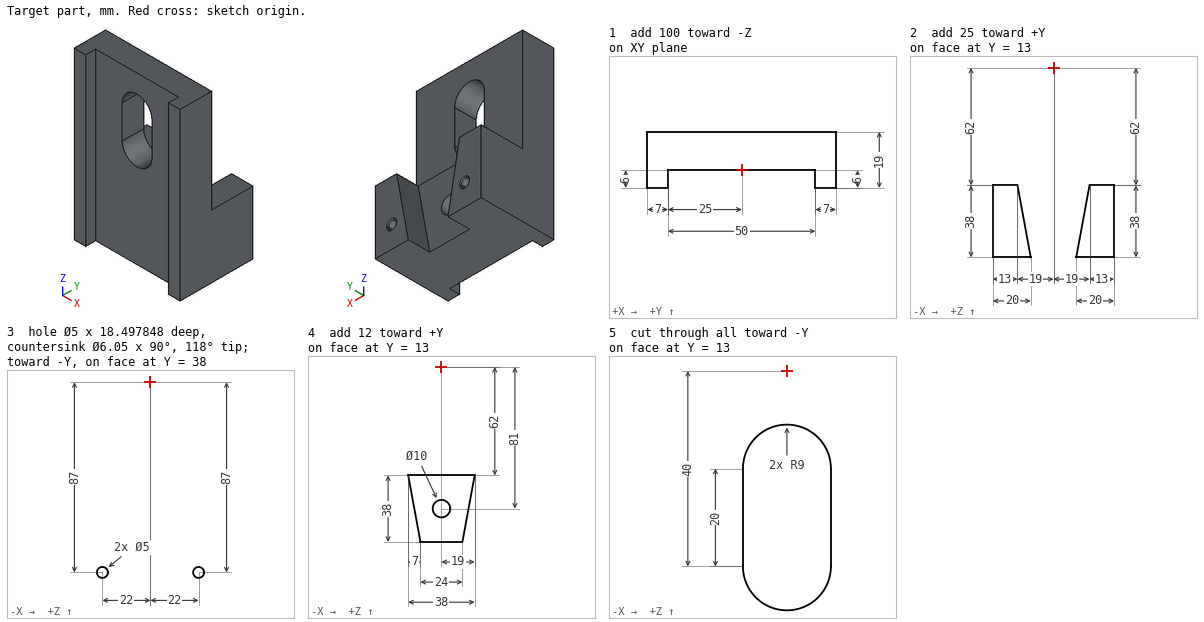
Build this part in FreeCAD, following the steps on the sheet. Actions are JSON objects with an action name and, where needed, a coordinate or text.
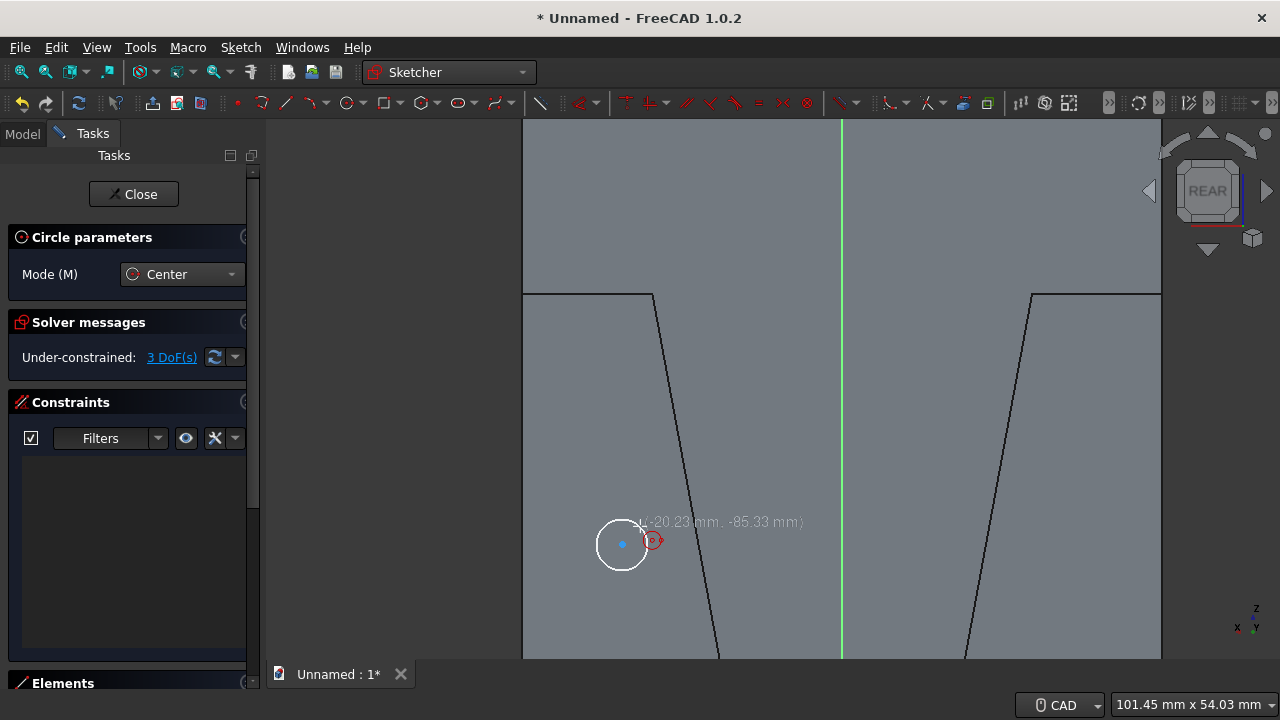
{"action": "left_click", "coordinate": [1062, 544]}
{"action": "left_click", "coordinate": [1080, 526]}
{"action": "key", "text": "Escape"}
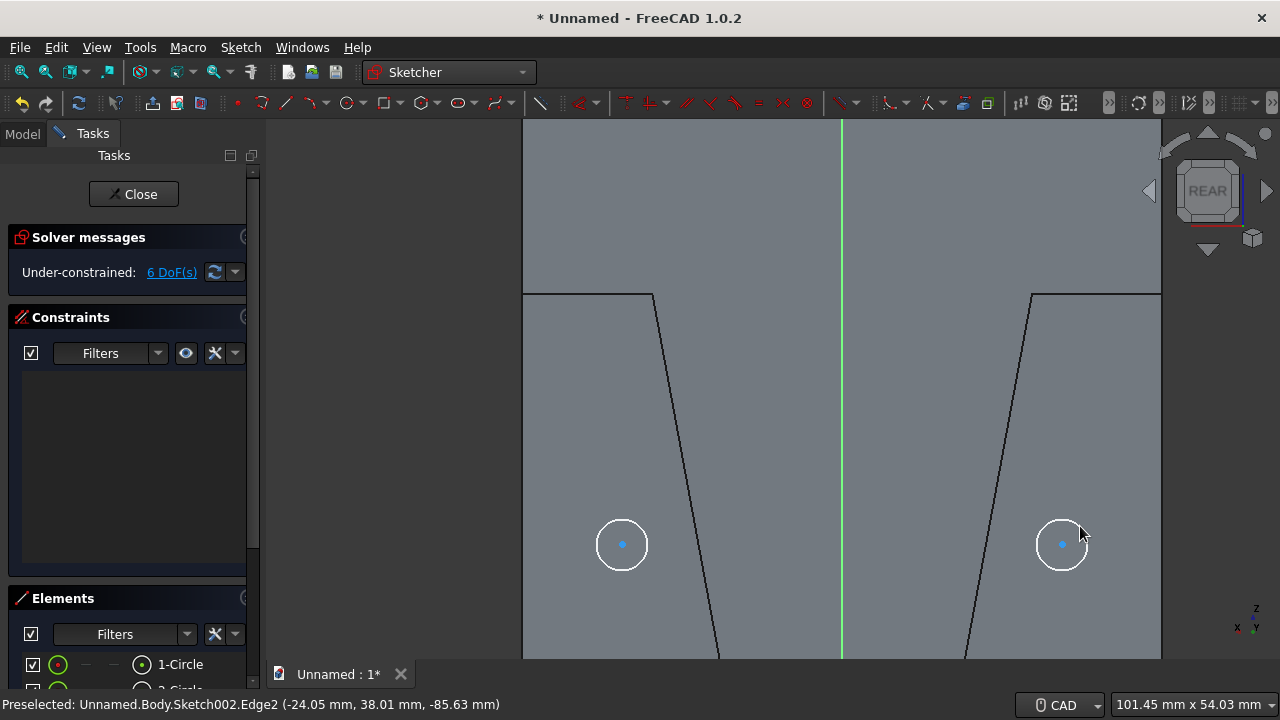
{"action": "left_click", "coordinate": [640, 527]}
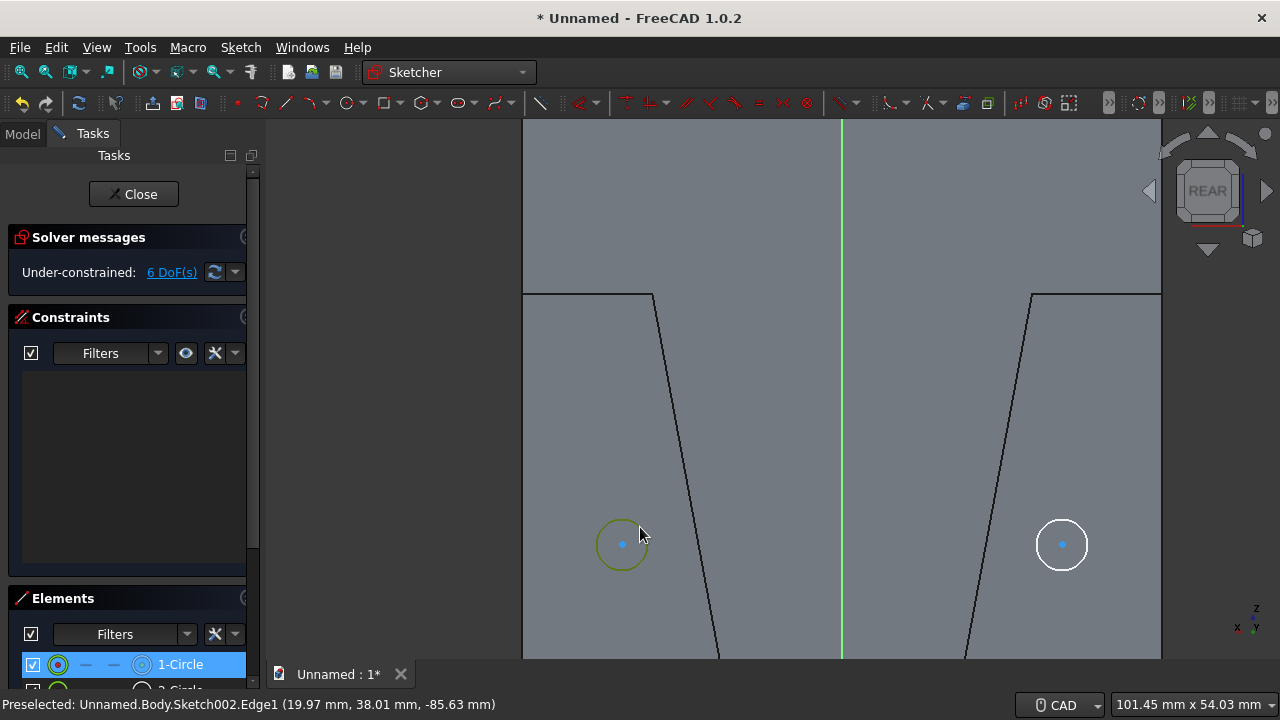
{"action": "left_click", "coordinate": [1080, 527]}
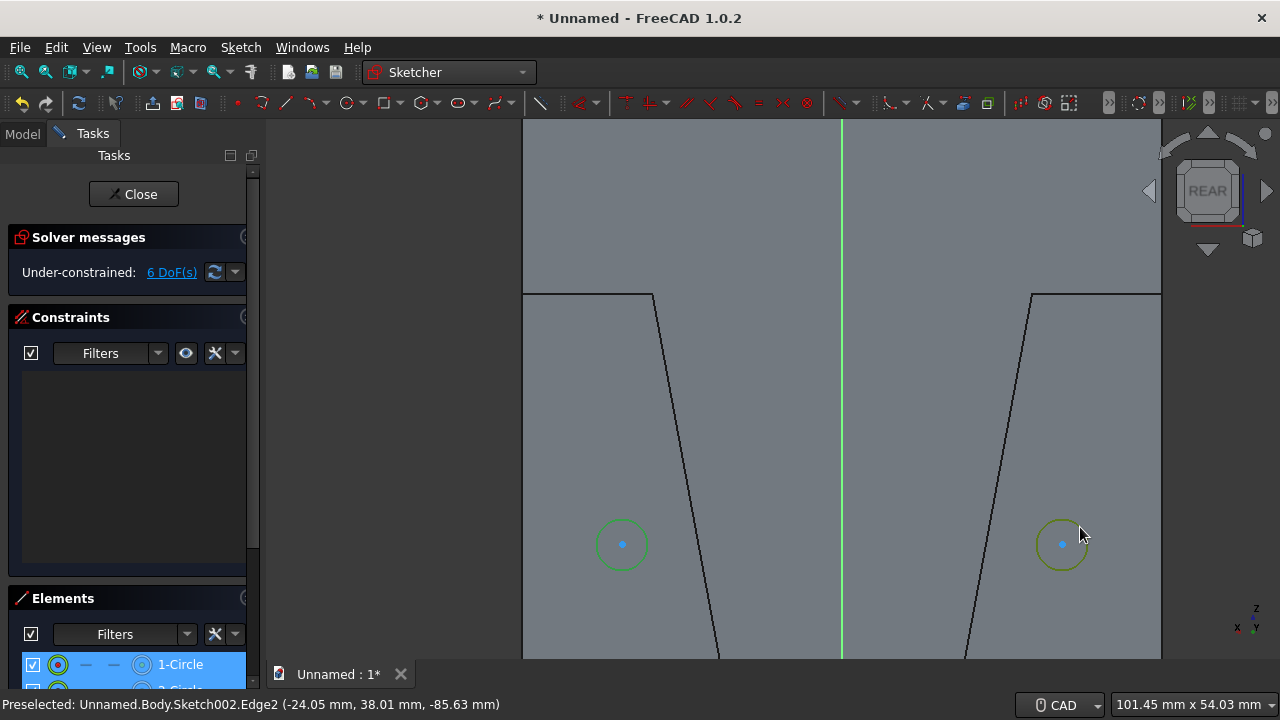
{"action": "key", "text": "e"}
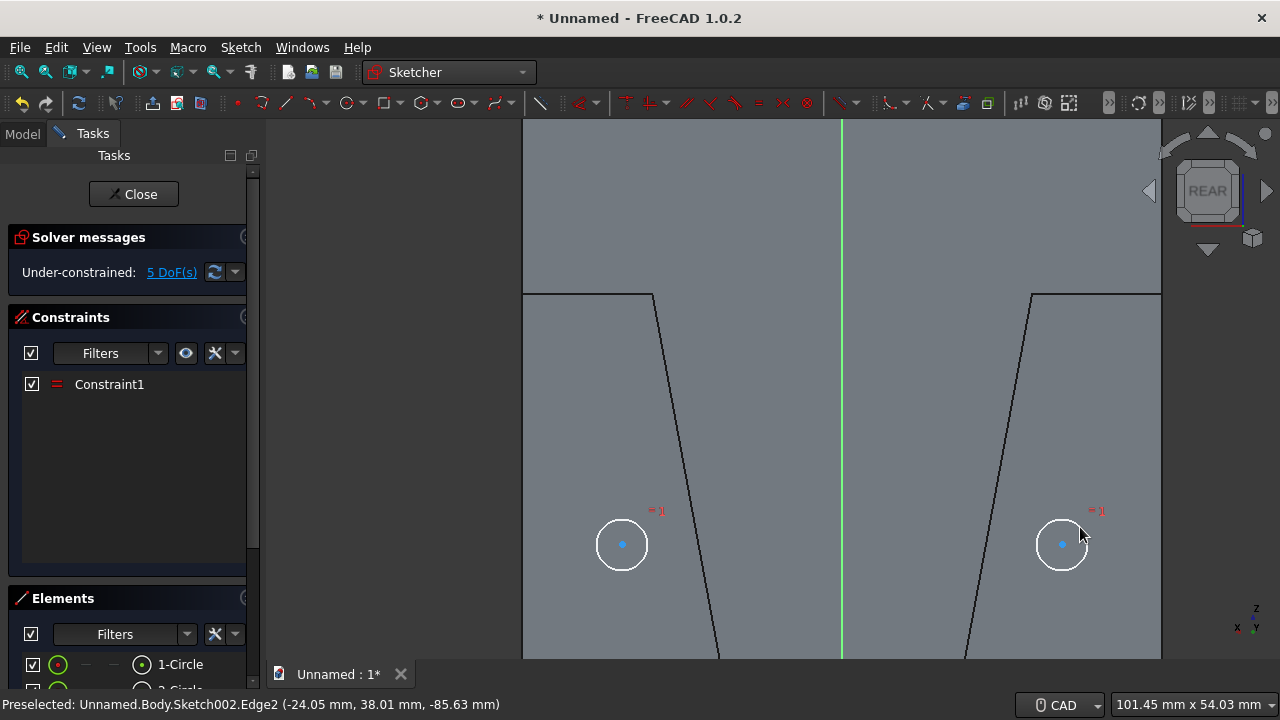
{"action": "key", "text": "d"}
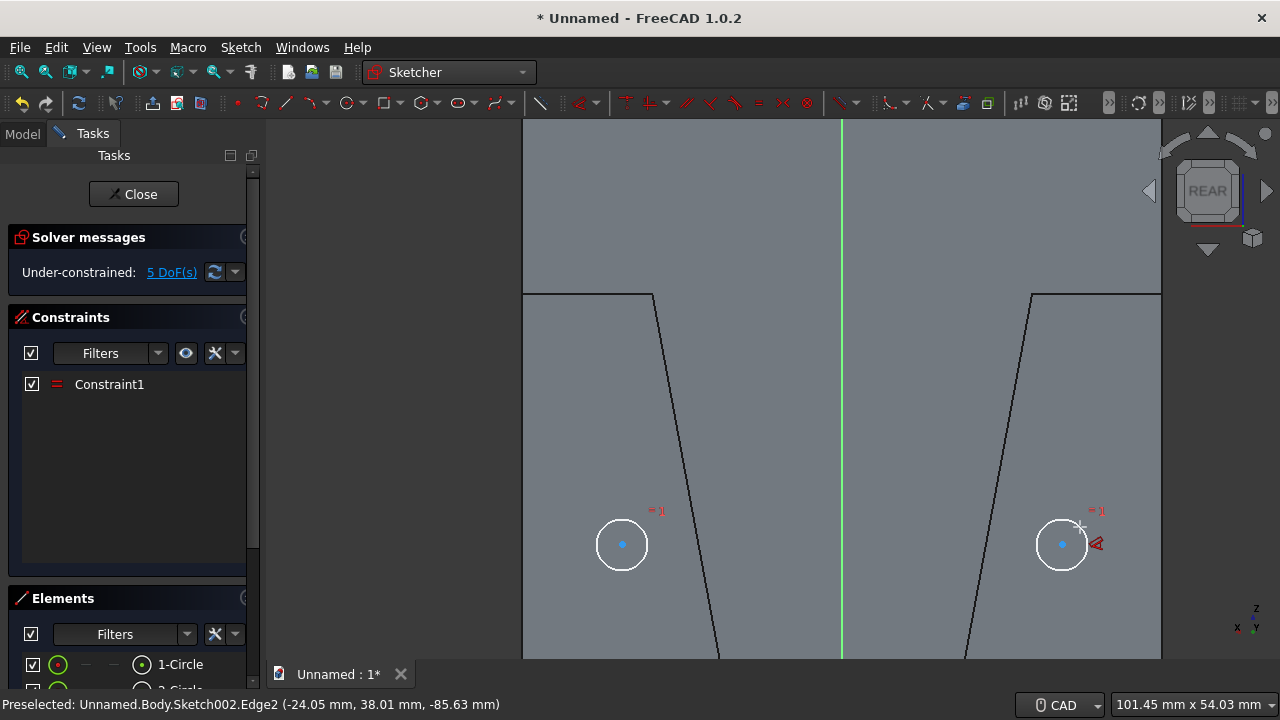
{"action": "left_click", "coordinate": [640, 527]}
{"action": "left_click", "coordinate": [663, 504]}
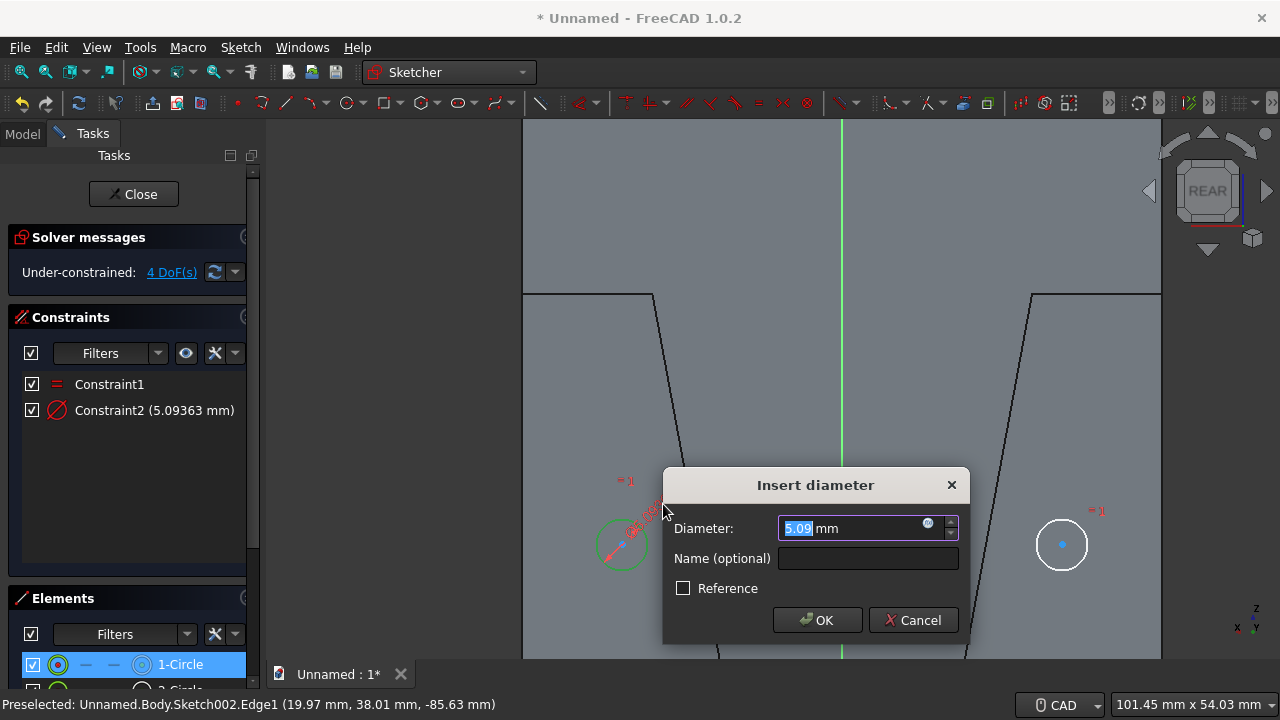
{"action": "type", "text": "5"}
{"action": "key", "text": "Return"}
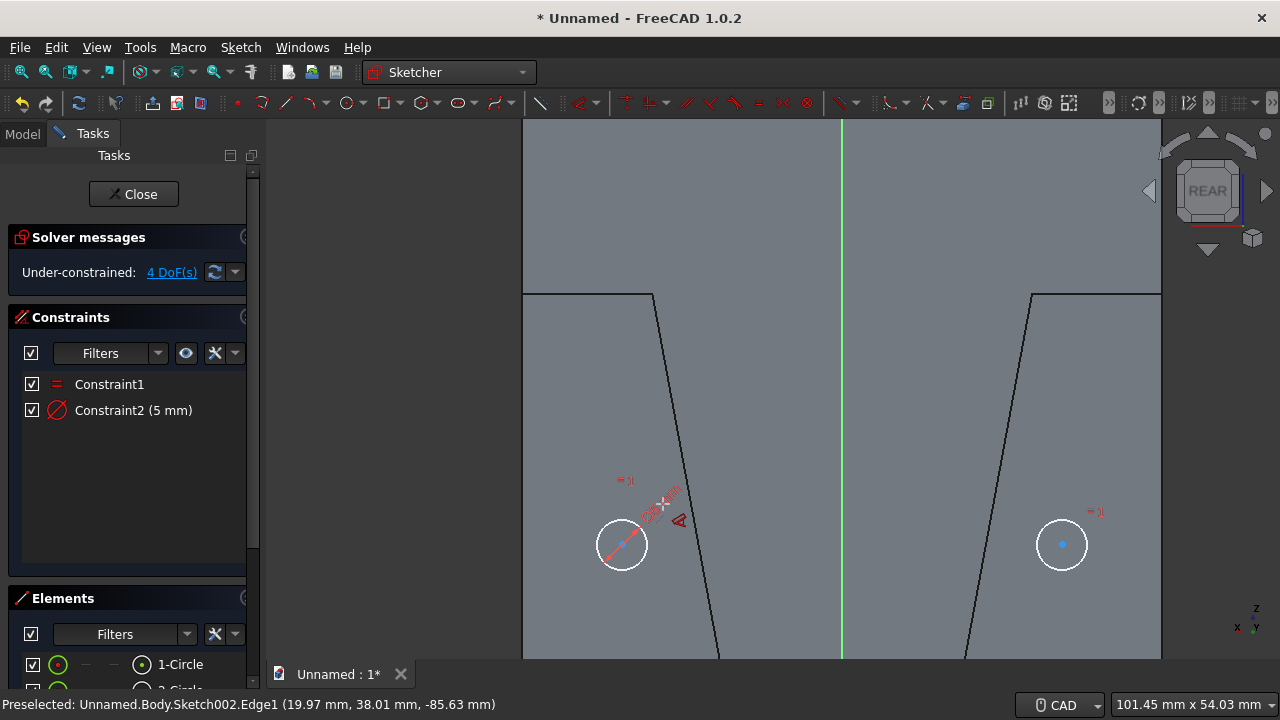
{"action": "left_click", "coordinate": [622, 545]}
{"action": "left_click", "coordinate": [732, 579]}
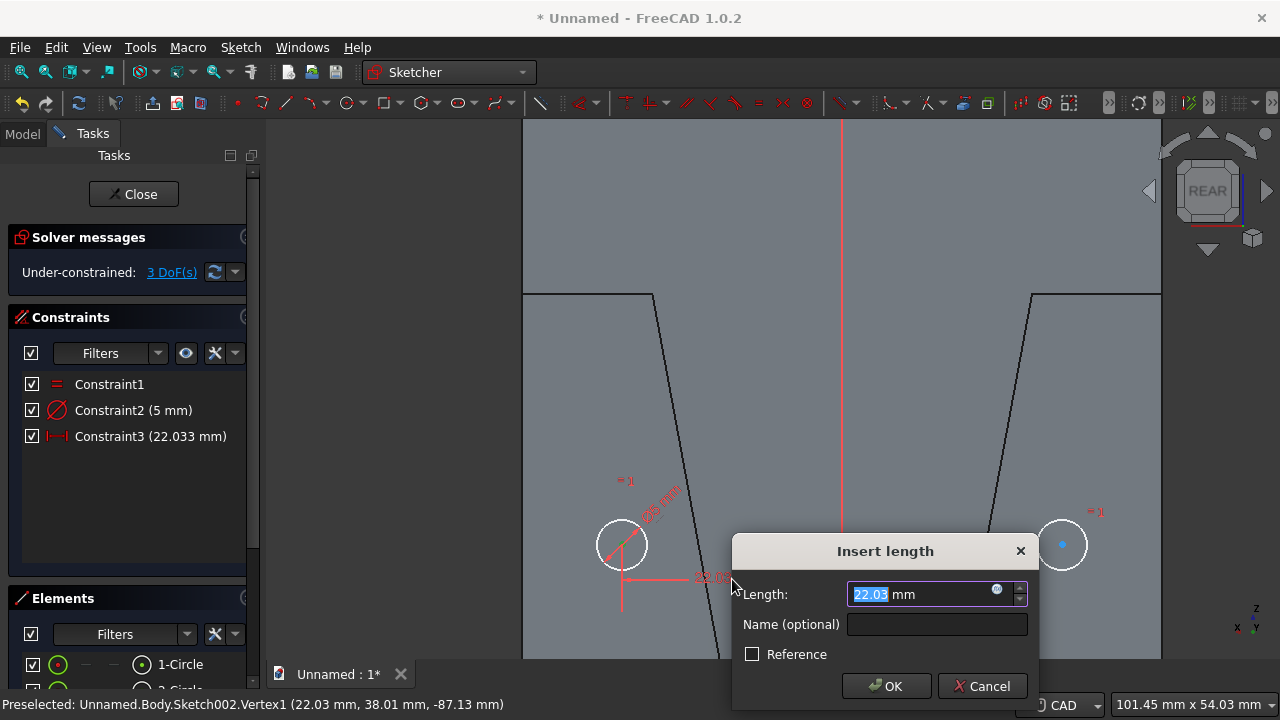
{"action": "type", "text": "22"}
{"action": "key", "text": "Return"}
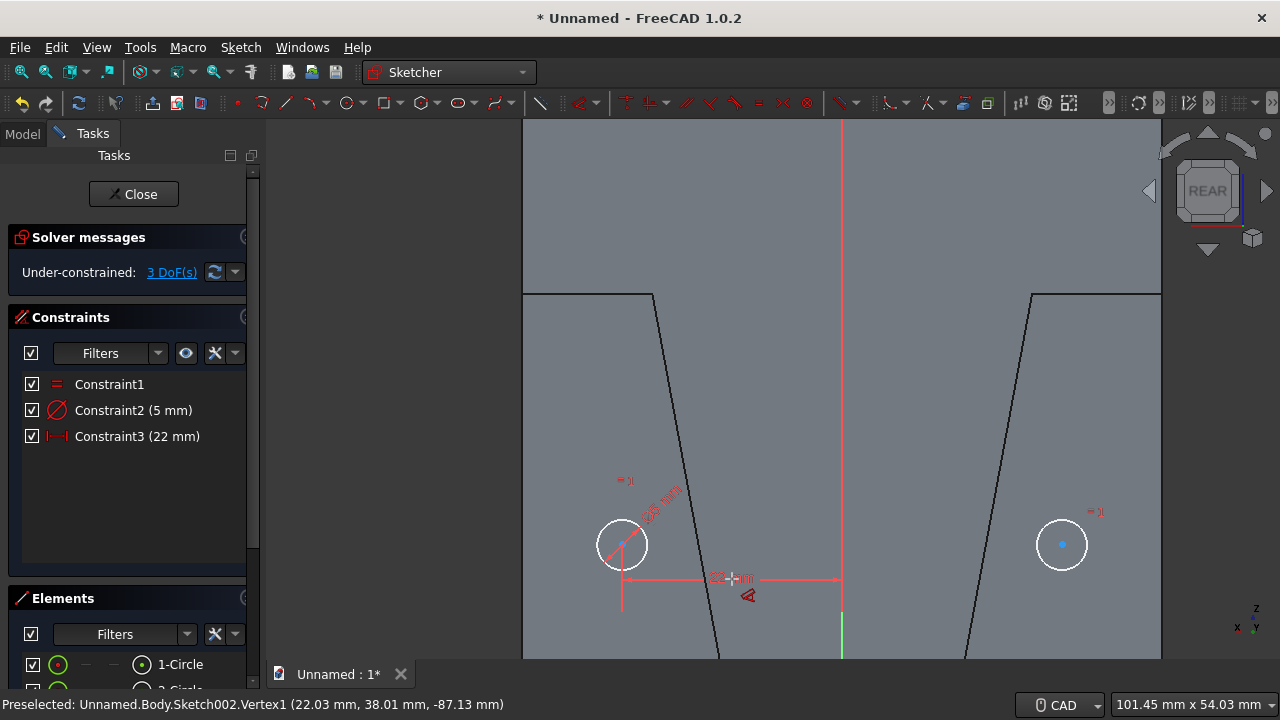
{"action": "left_click", "coordinate": [622, 545]}
{"action": "left_click", "coordinate": [588, 346]}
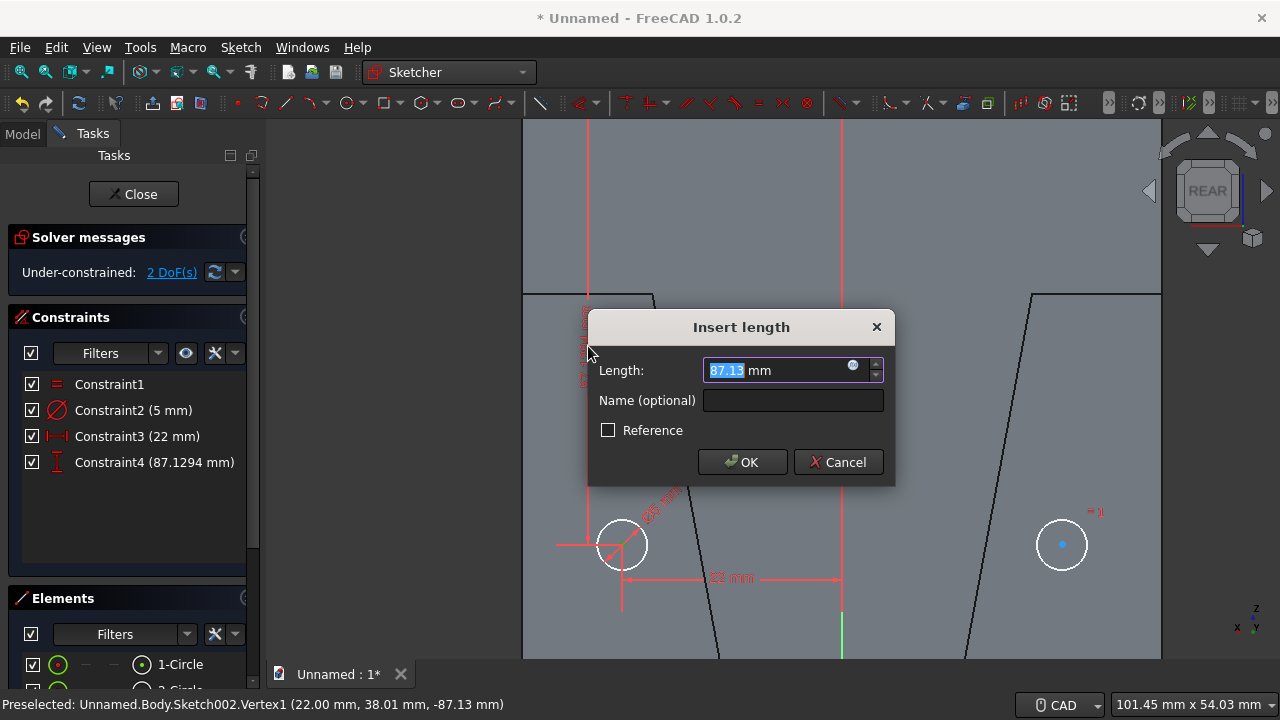
{"action": "type", "text": "87"}
{"action": "key", "text": "Return"}